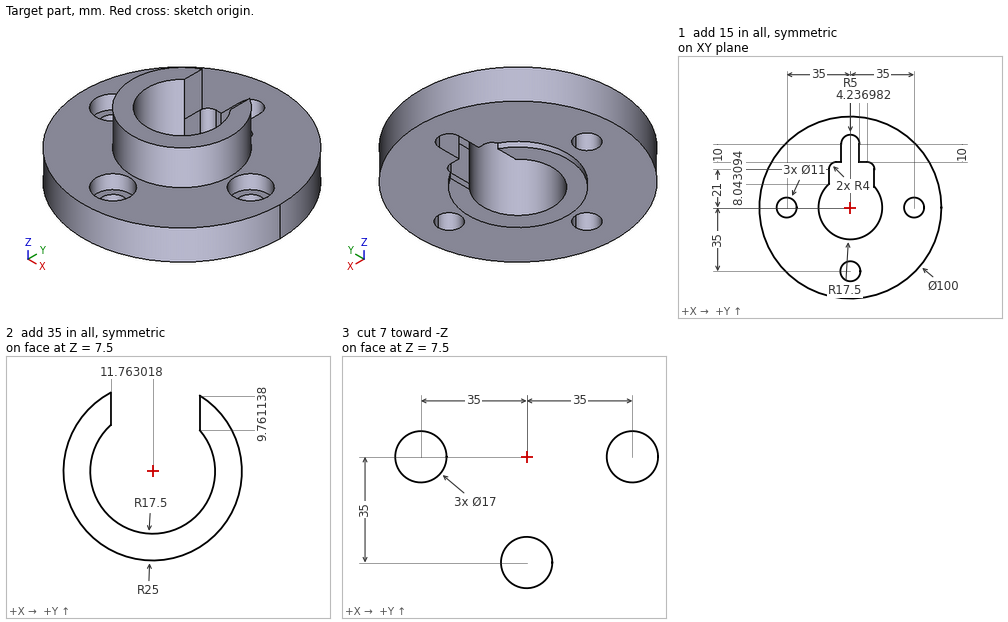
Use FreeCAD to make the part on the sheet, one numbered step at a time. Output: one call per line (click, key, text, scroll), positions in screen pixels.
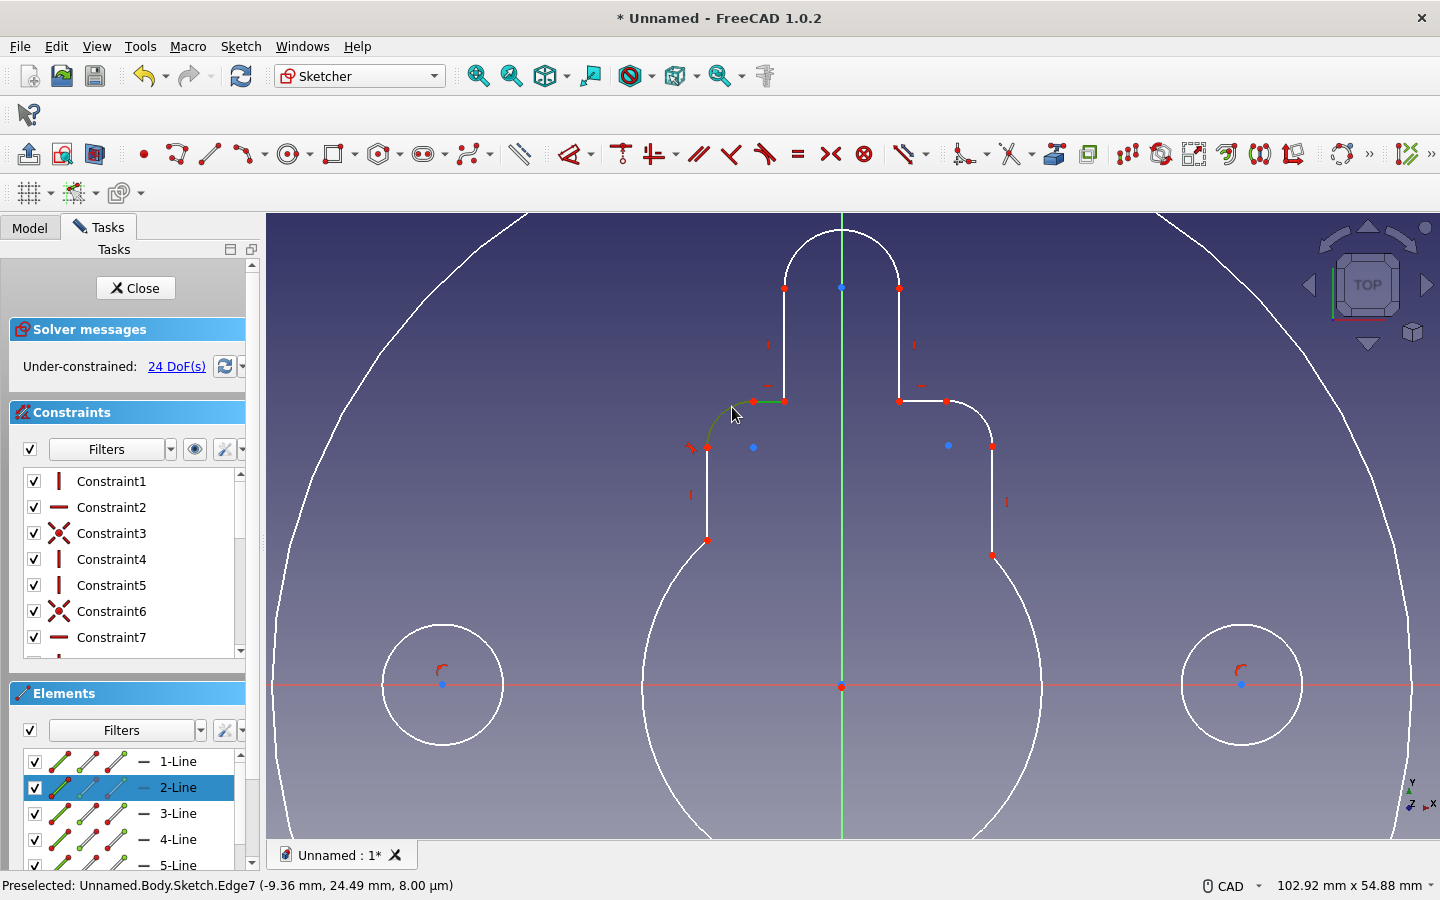
click(765, 154)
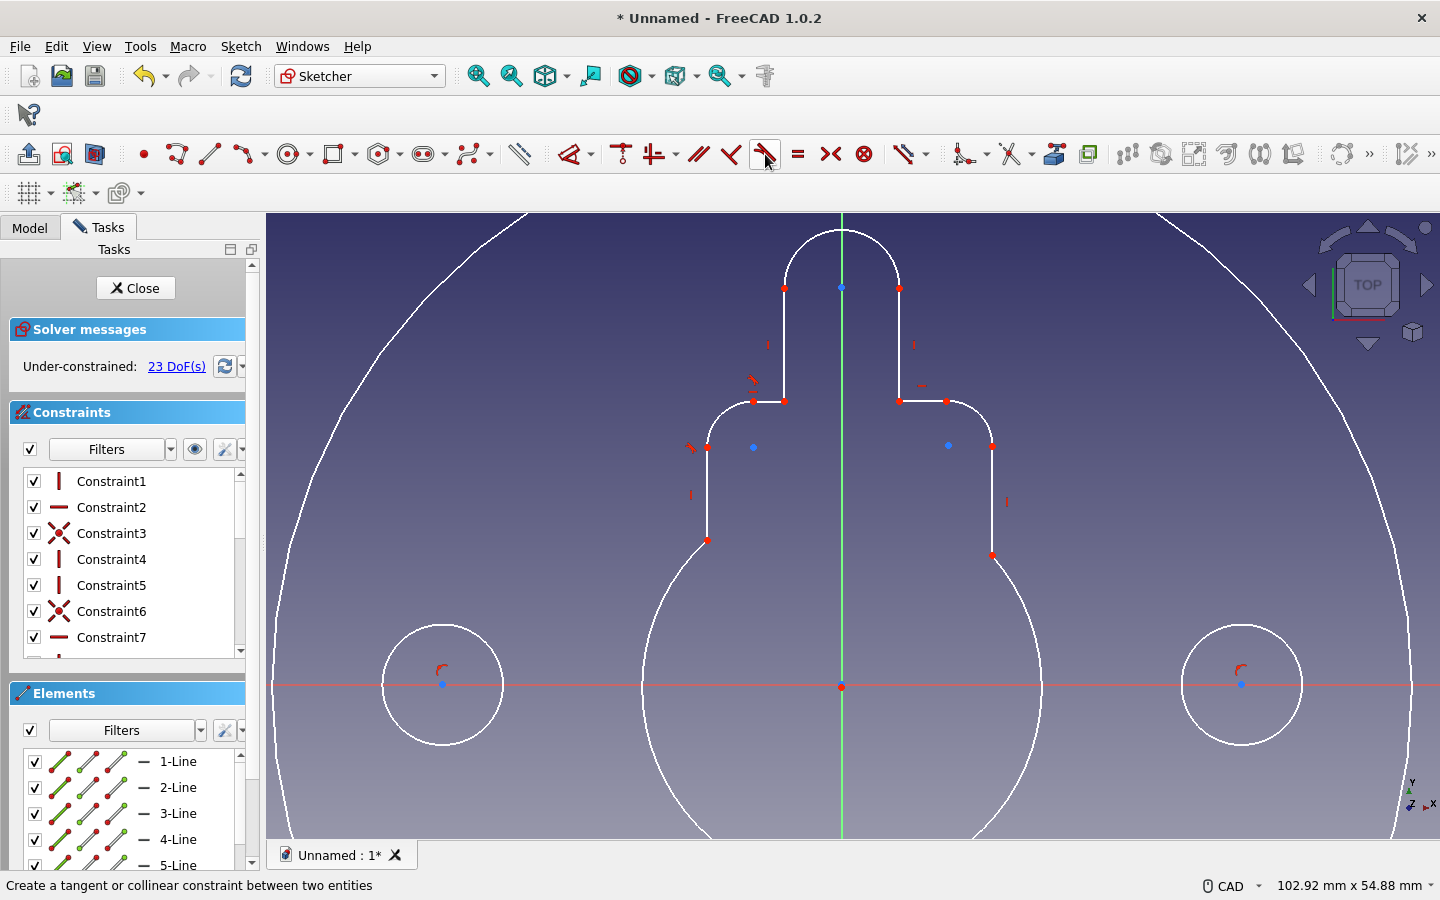
click(784, 368)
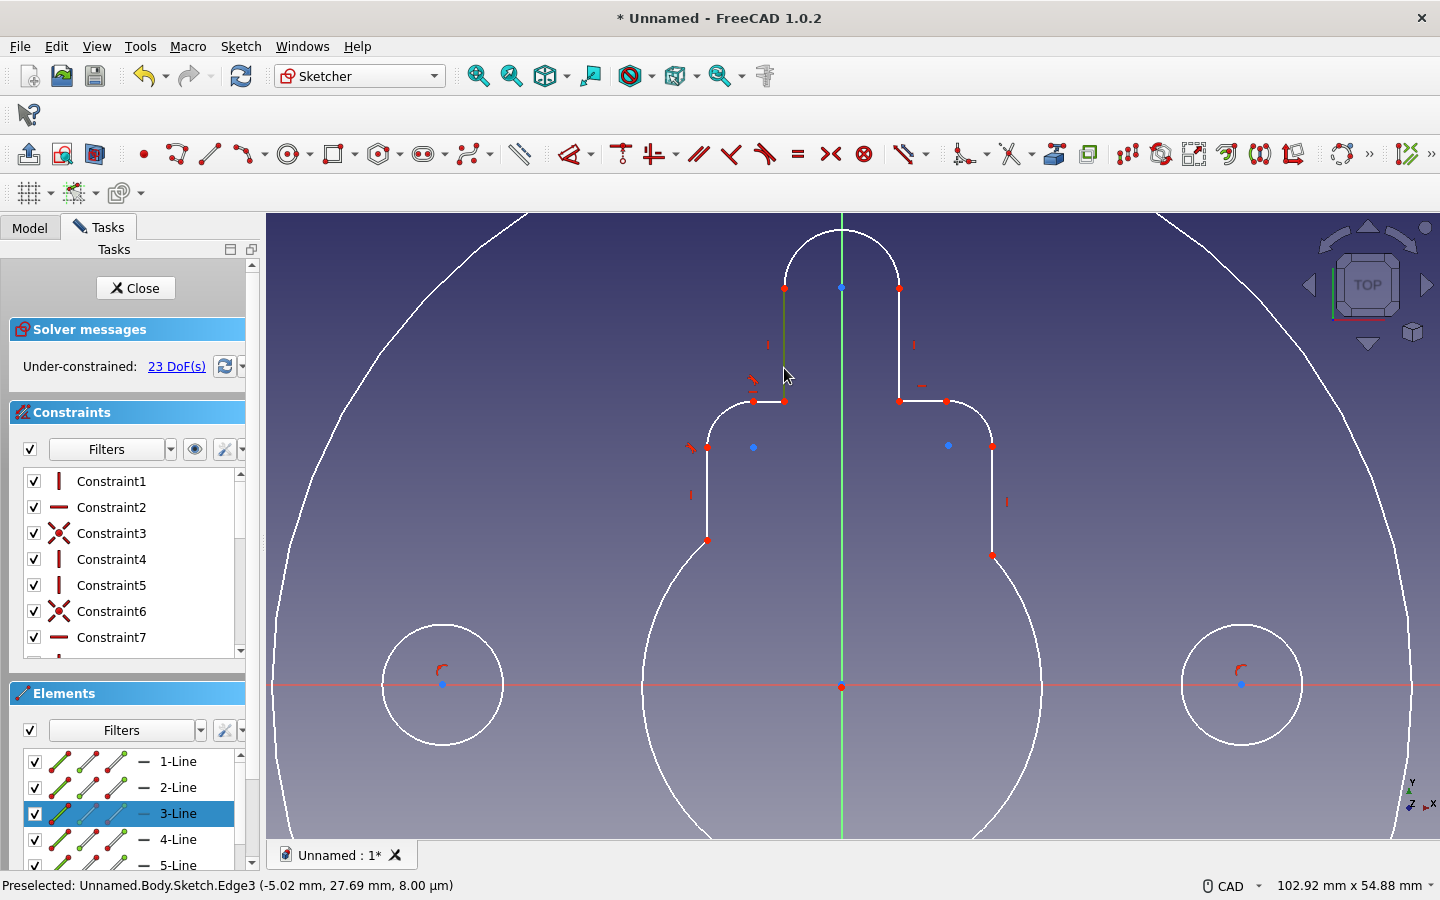
click(876, 241)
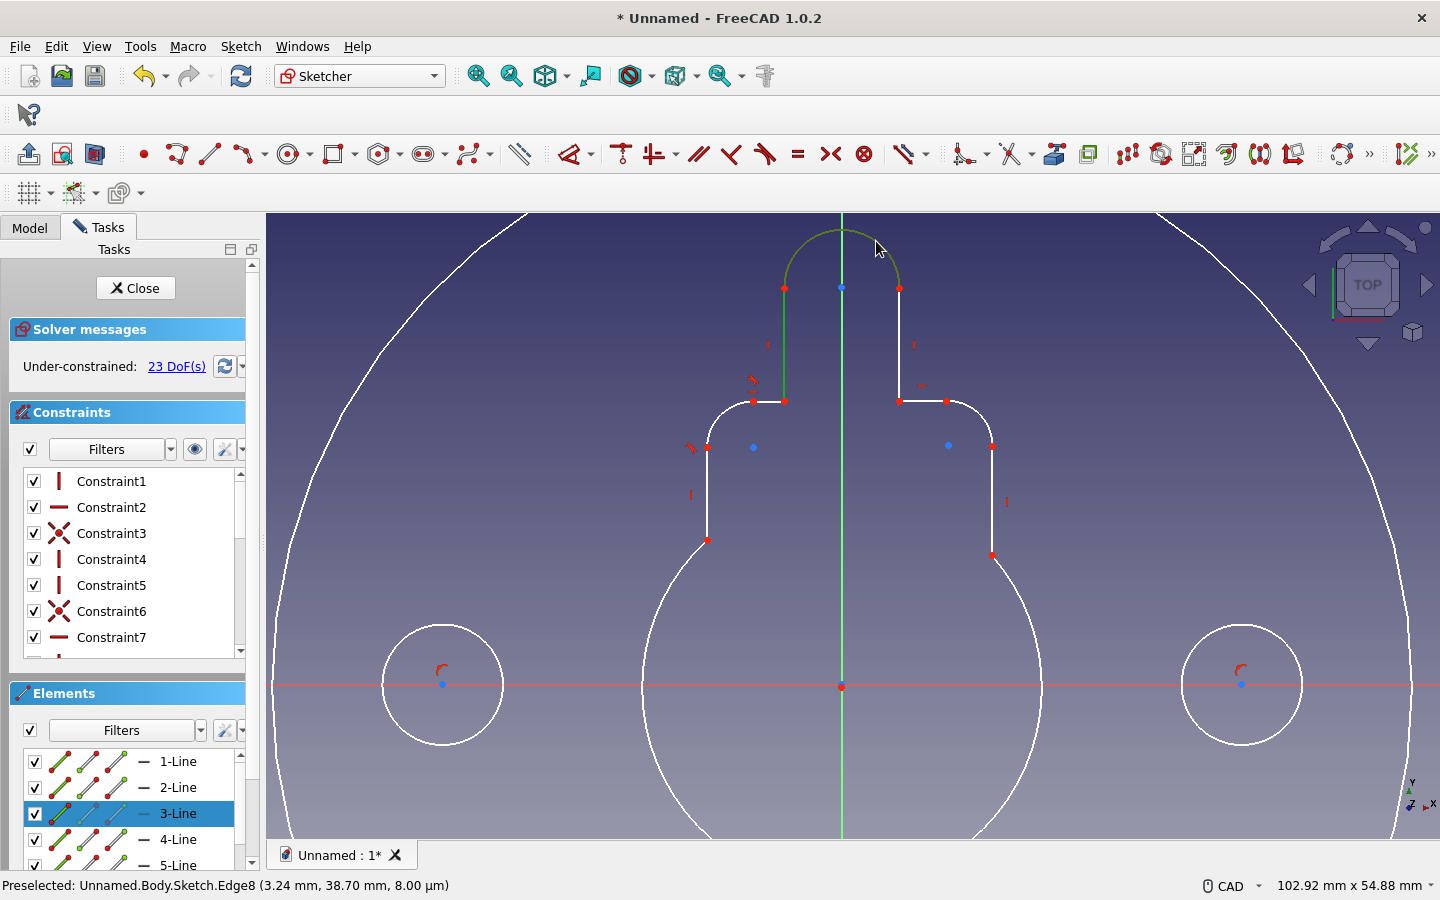
key(t)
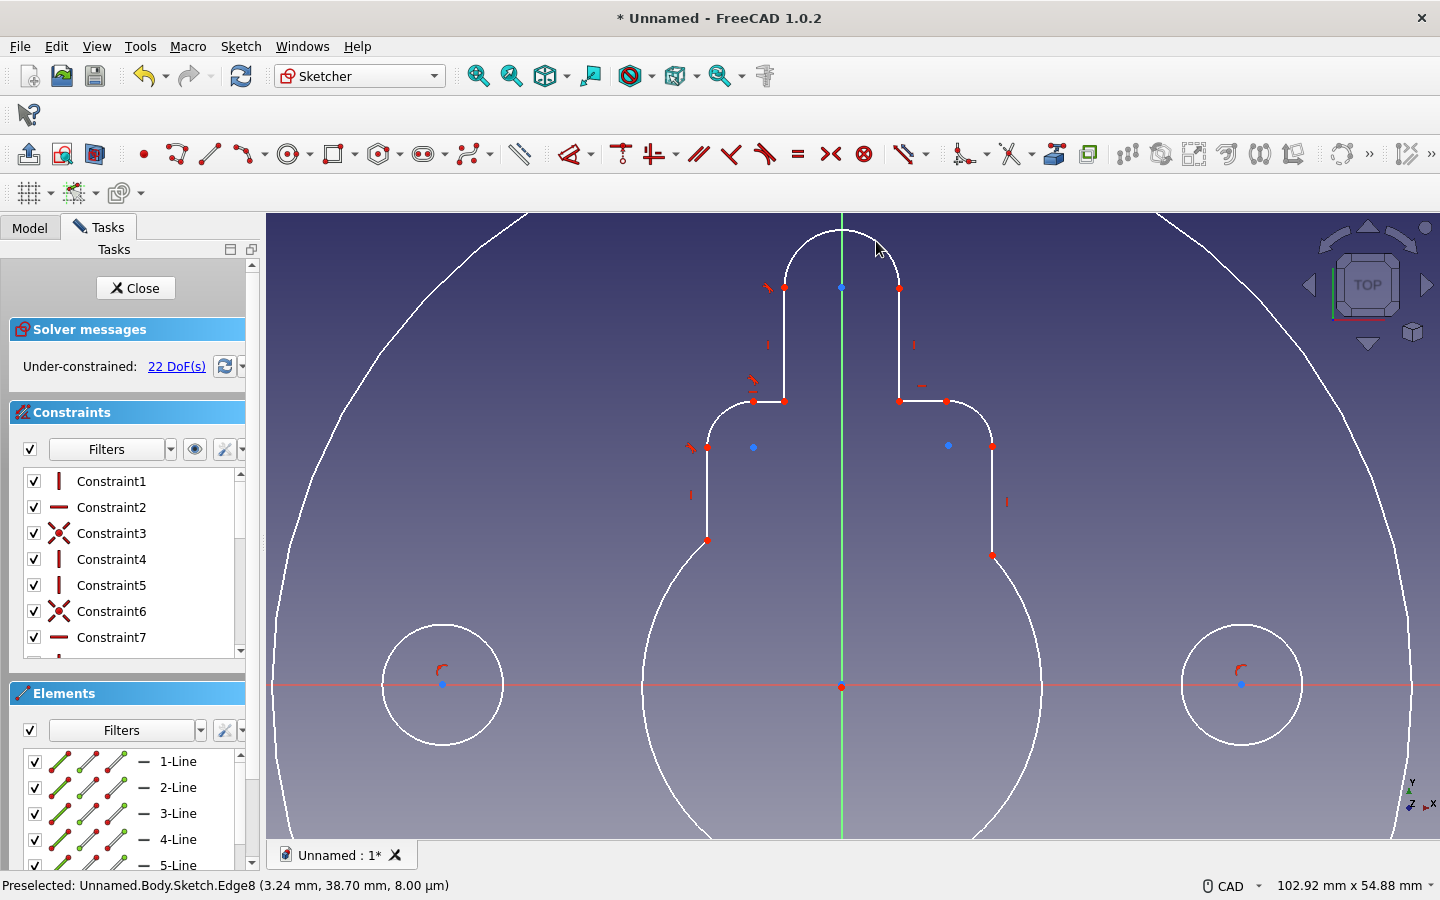
click(899, 322)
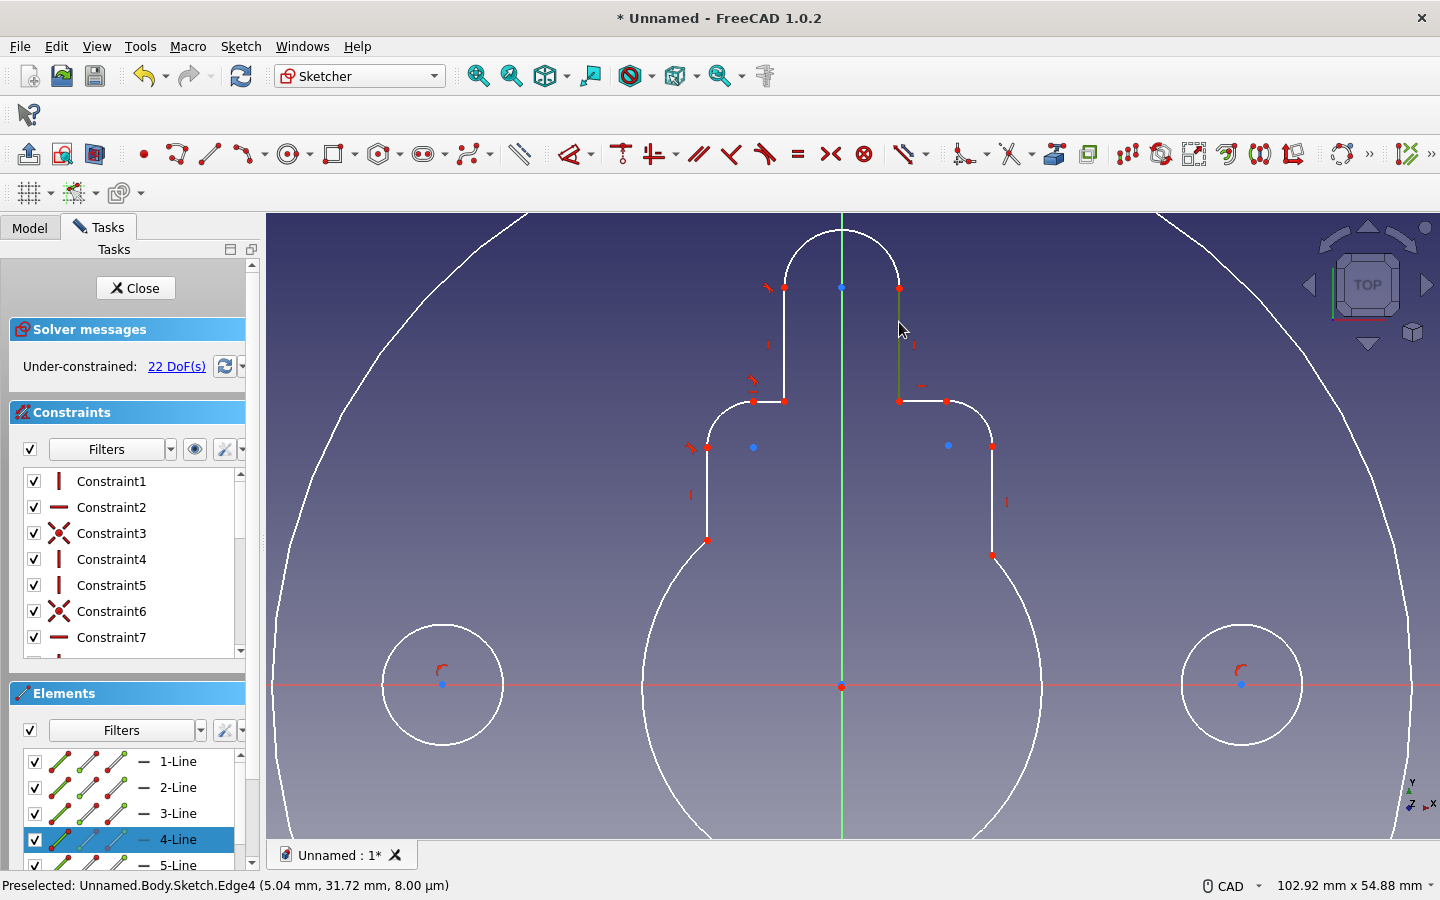
click(876, 241)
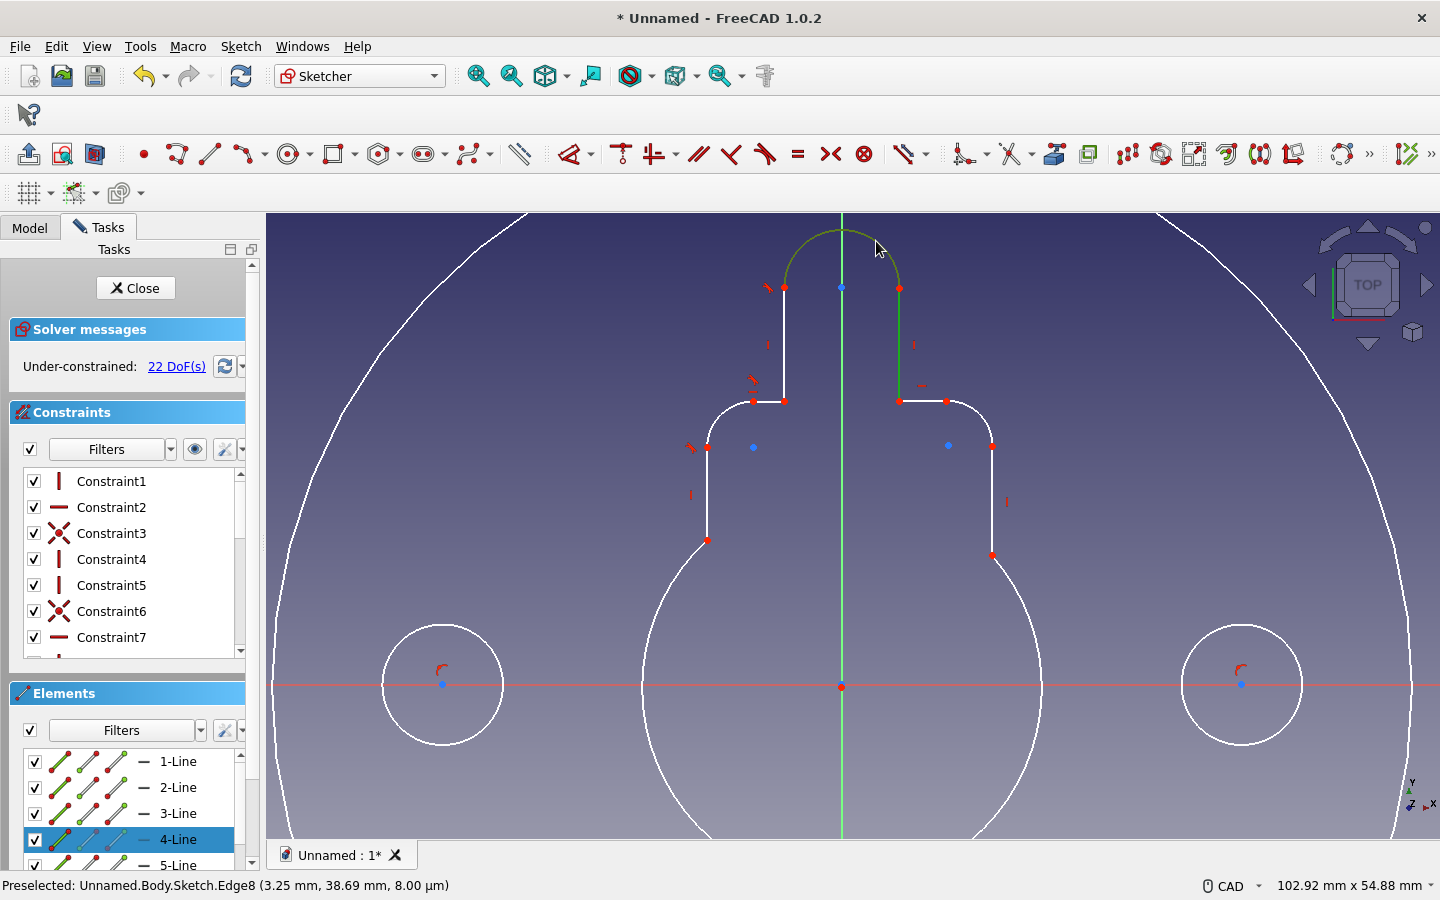
key(t)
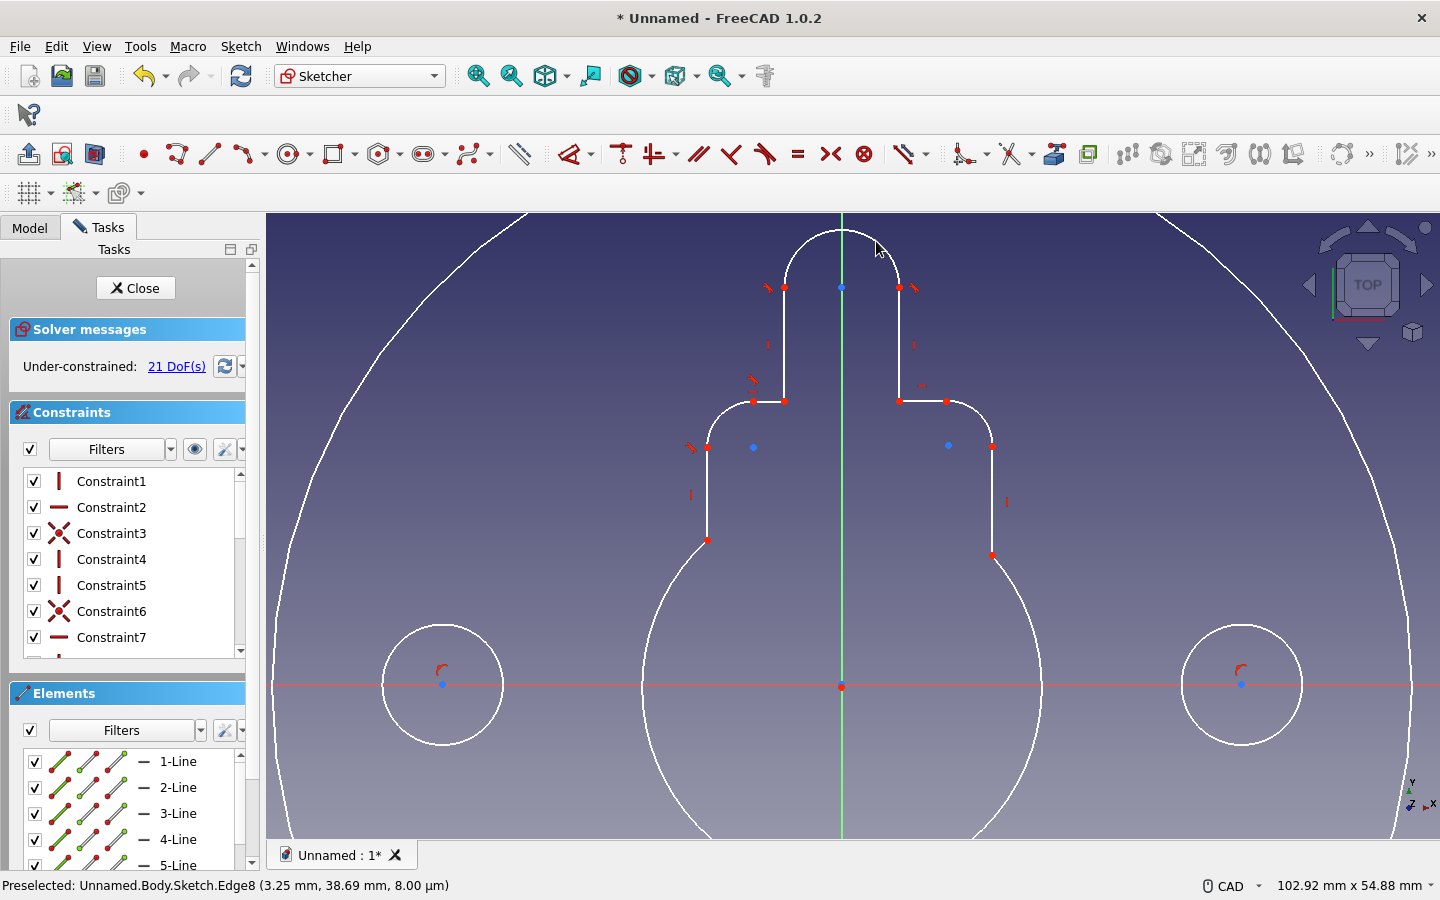
click(913, 401)